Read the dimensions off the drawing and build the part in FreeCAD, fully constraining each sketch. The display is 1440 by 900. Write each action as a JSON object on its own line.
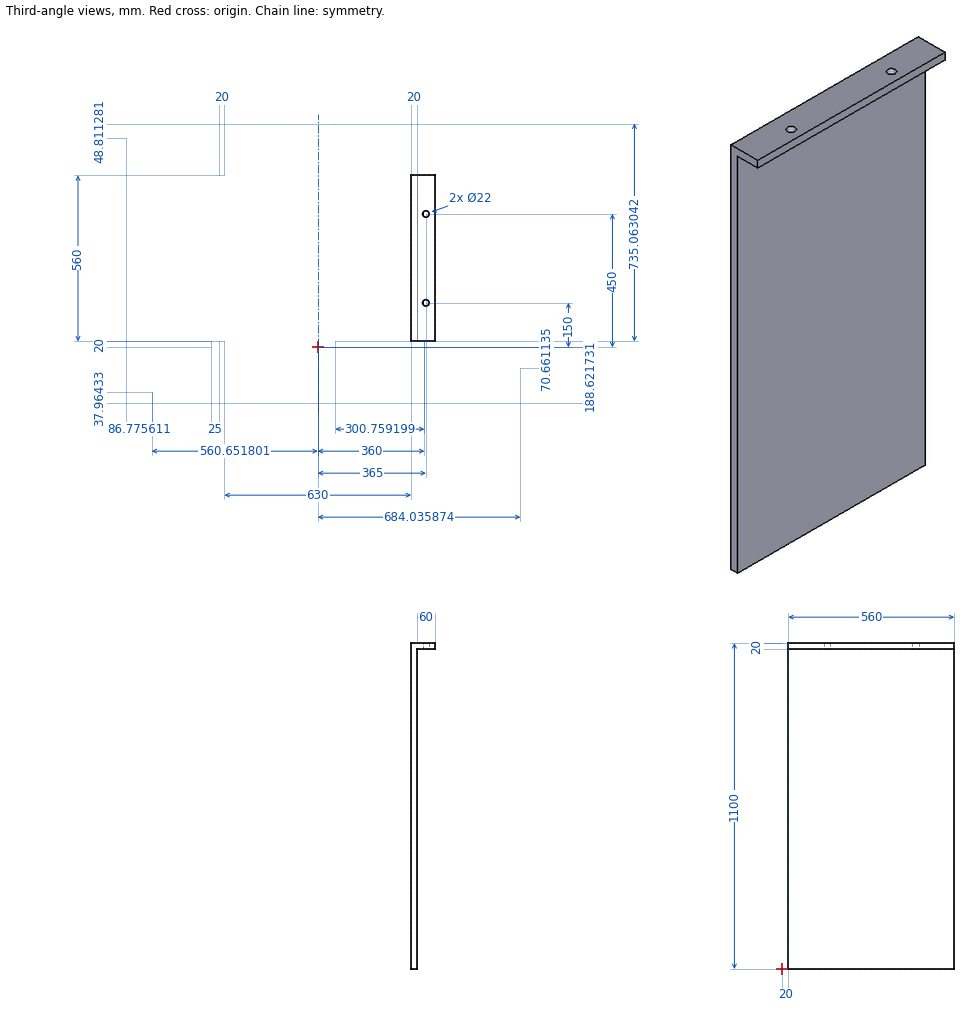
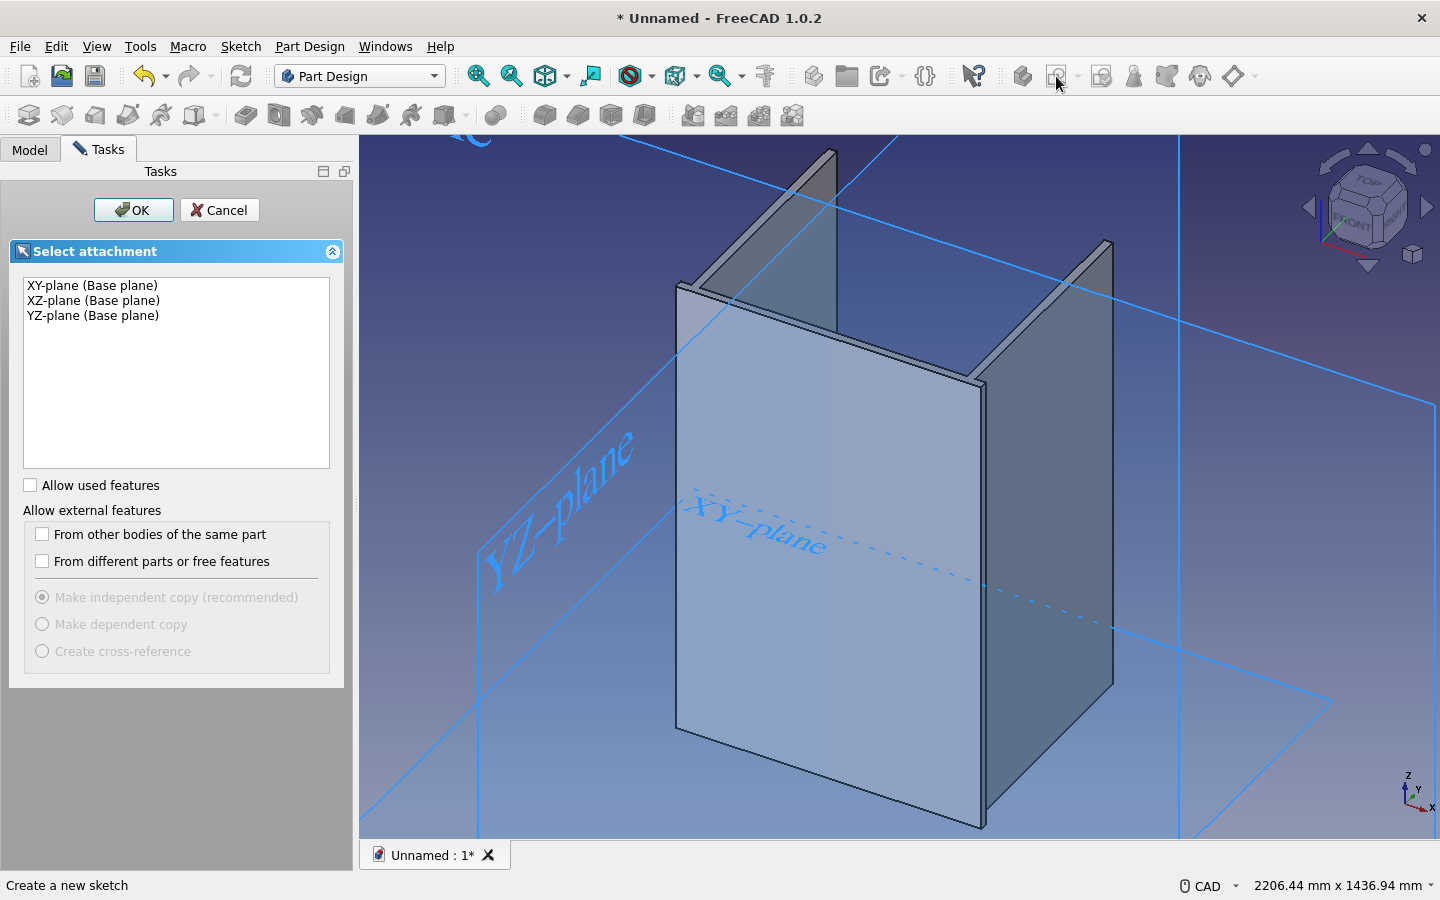
{"action": "left_click", "coordinate": [84, 286]}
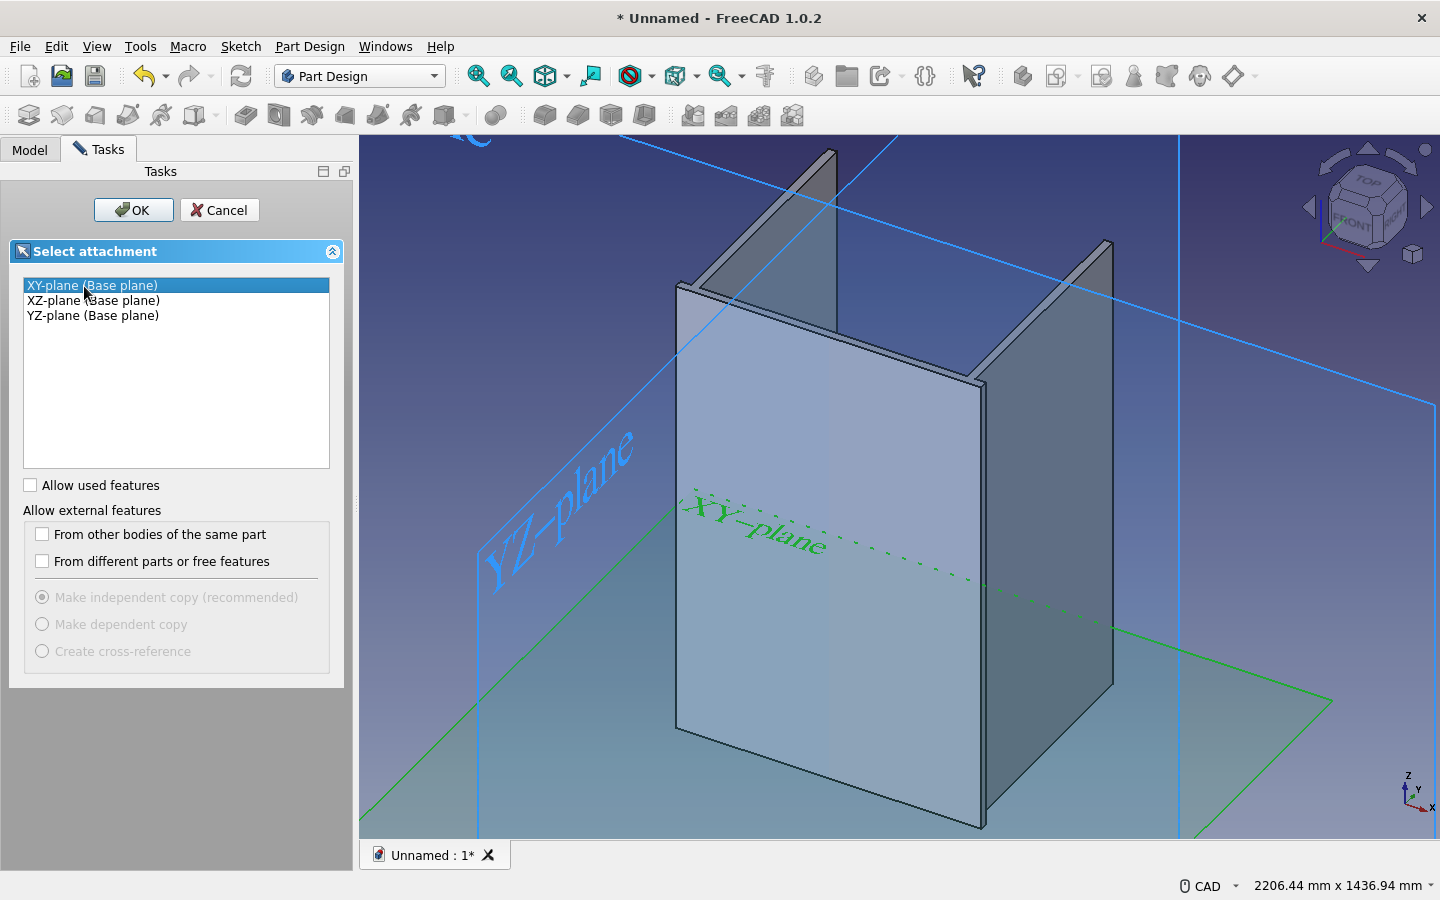
{"action": "left_click", "coordinate": [134, 210]}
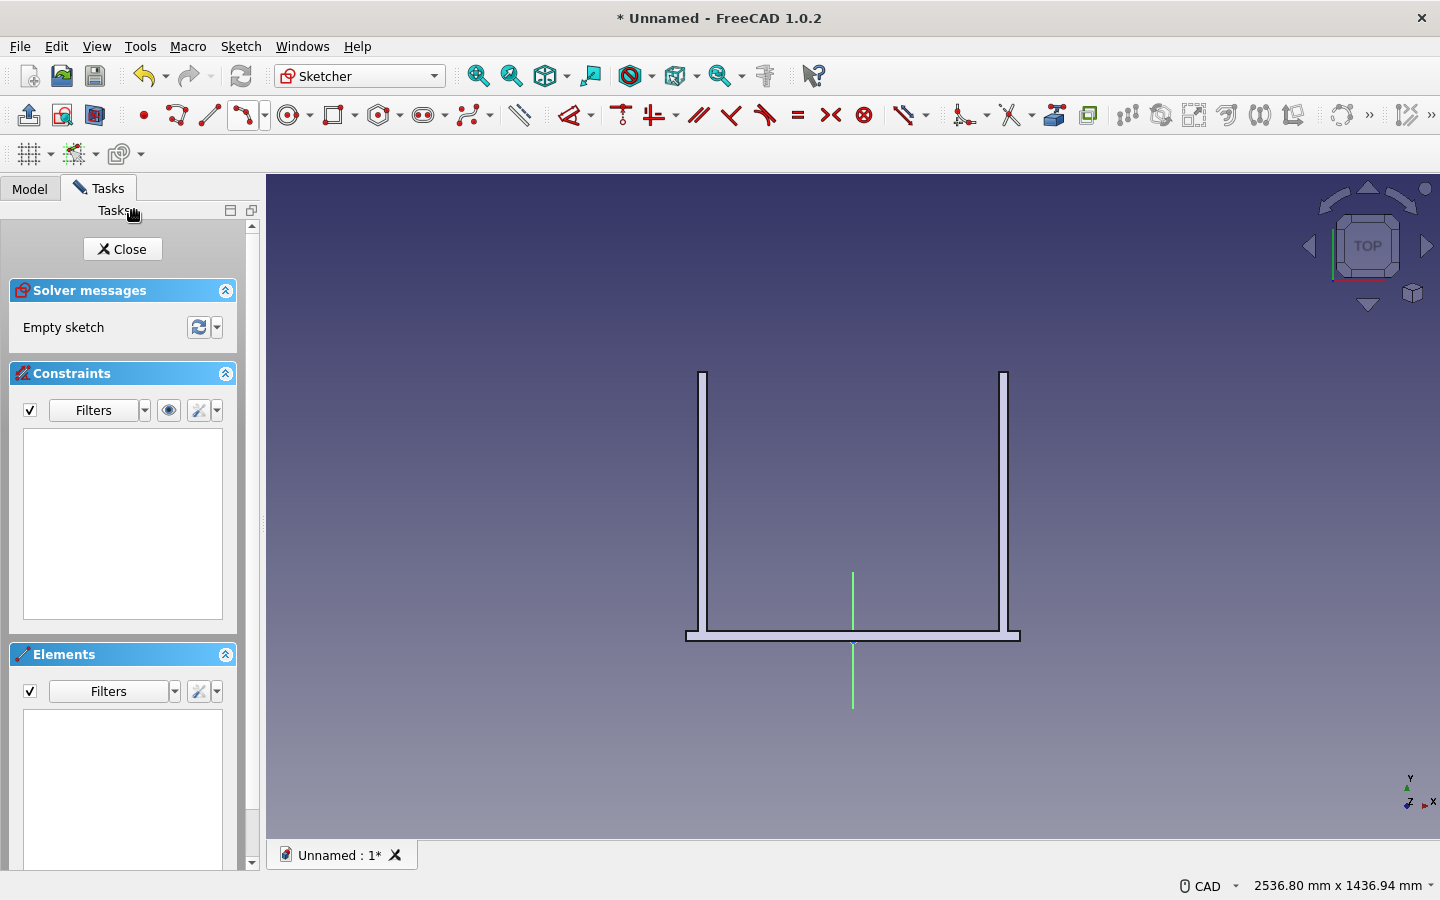
{"action": "left_click", "coordinate": [95, 116]}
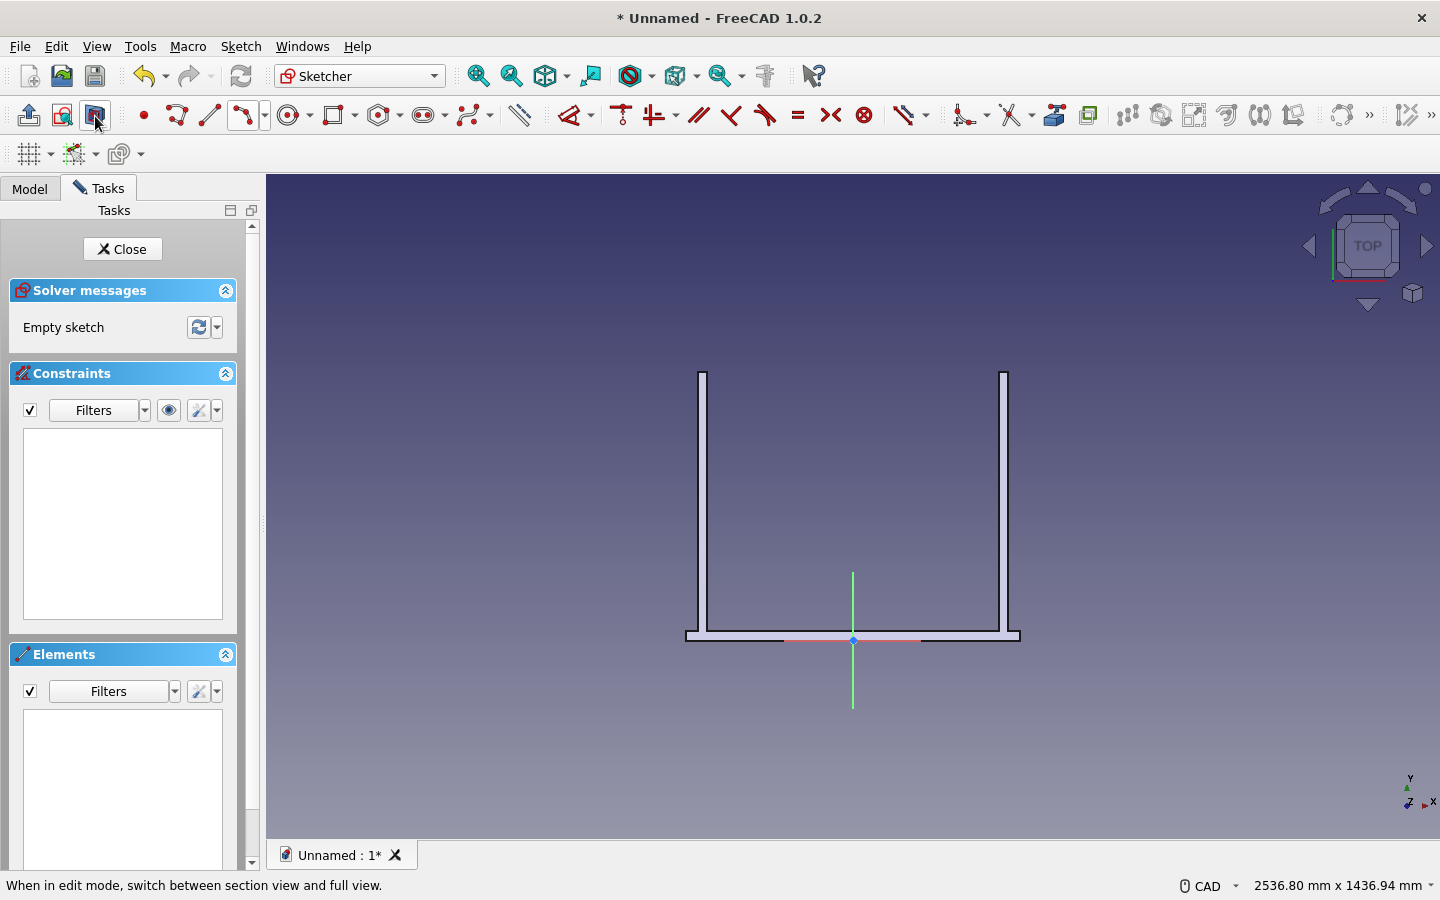
{"action": "left_click", "coordinate": [177, 116]}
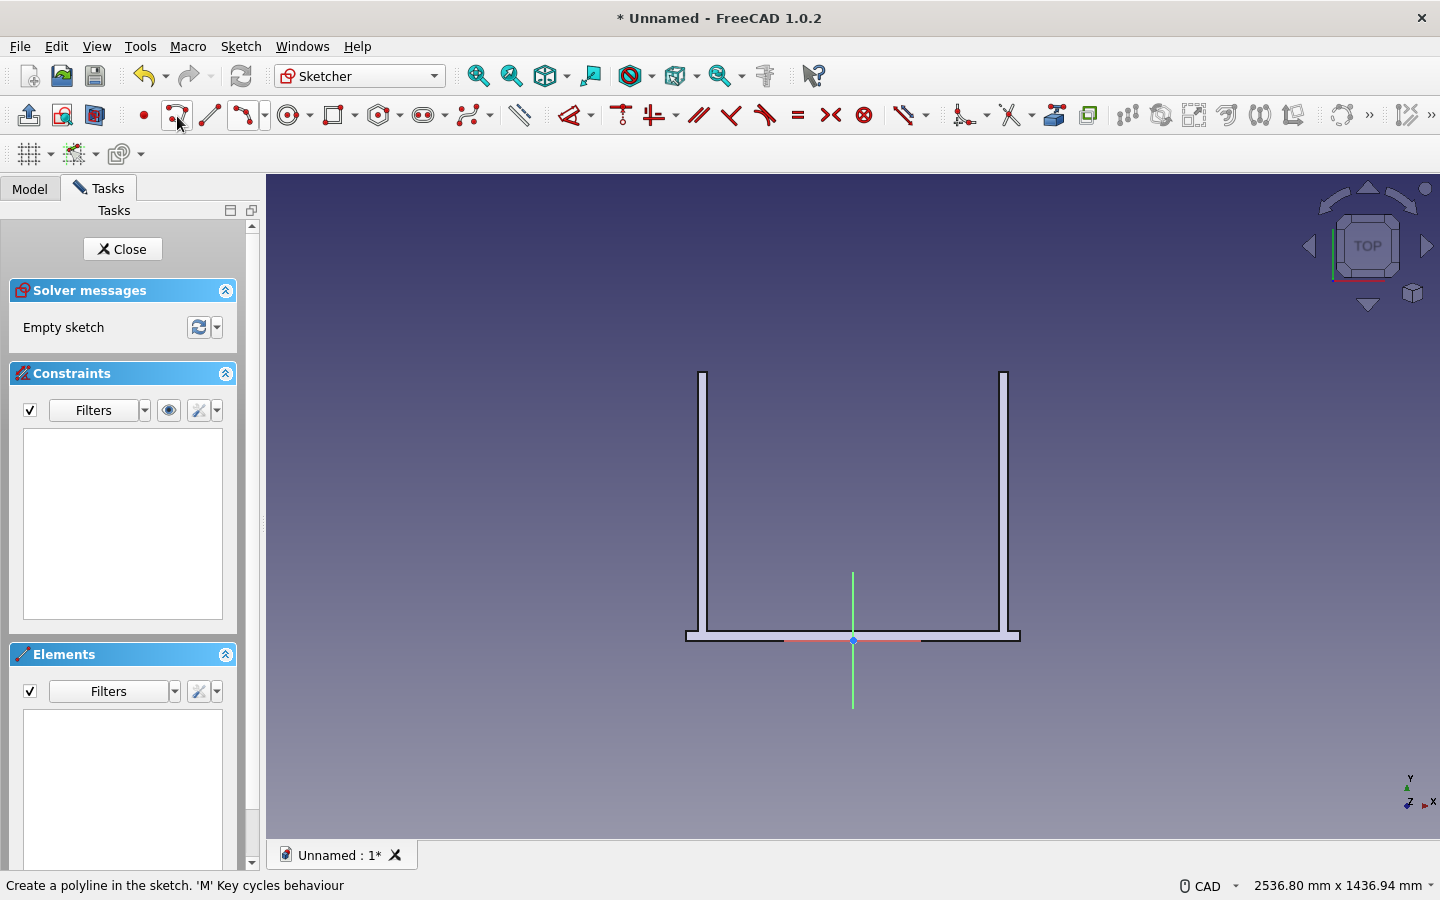
{"action": "scroll", "coordinate": [880, 631], "scroll_direction": "up", "scroll_amount": 3}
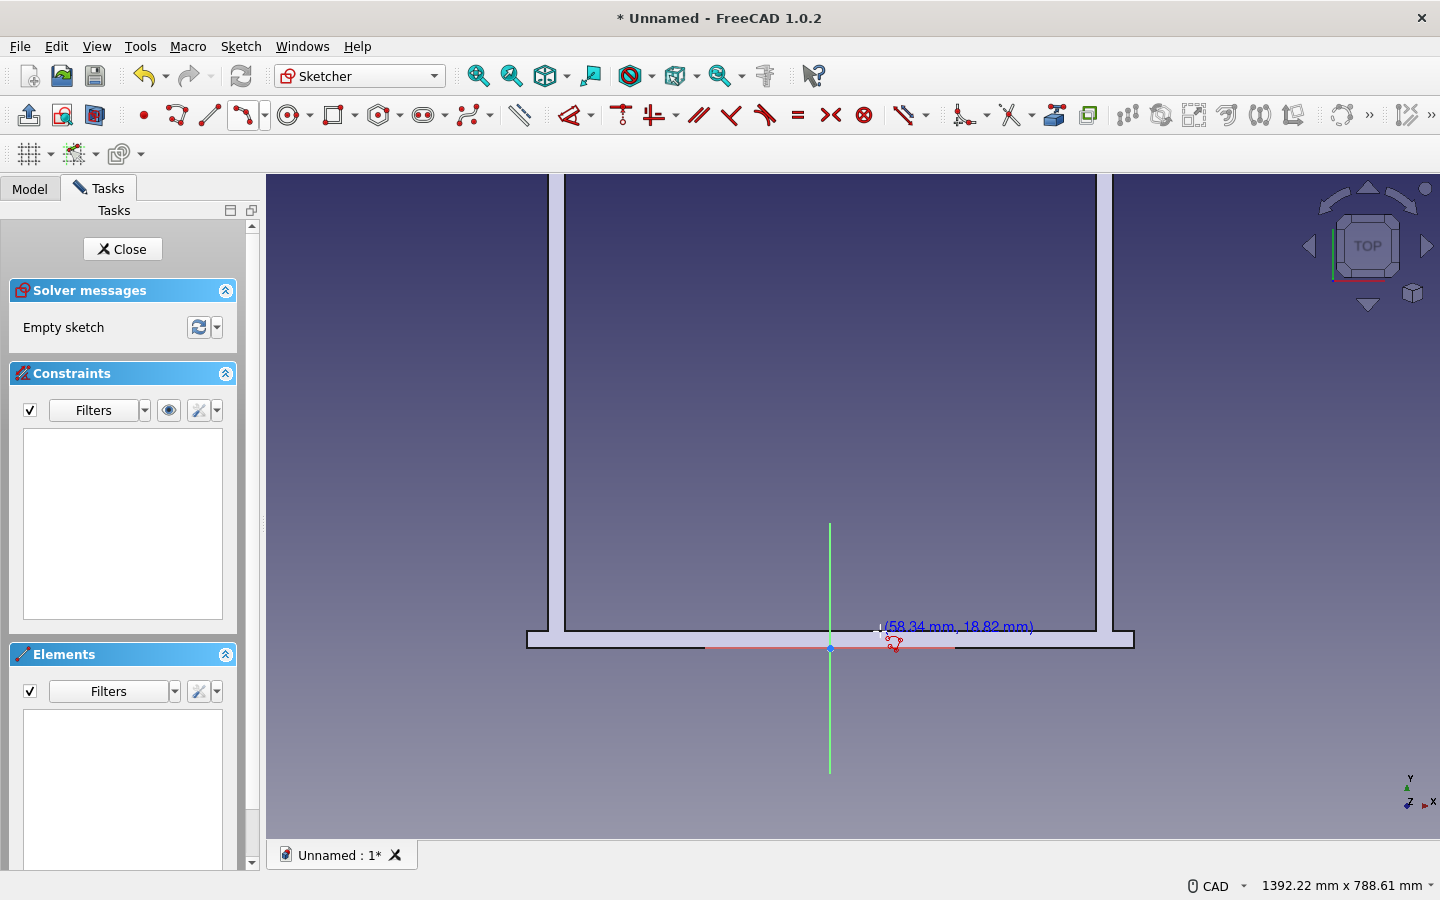
{"action": "left_click", "coordinate": [880, 631]}
{"action": "left_click", "coordinate": [1134, 631]}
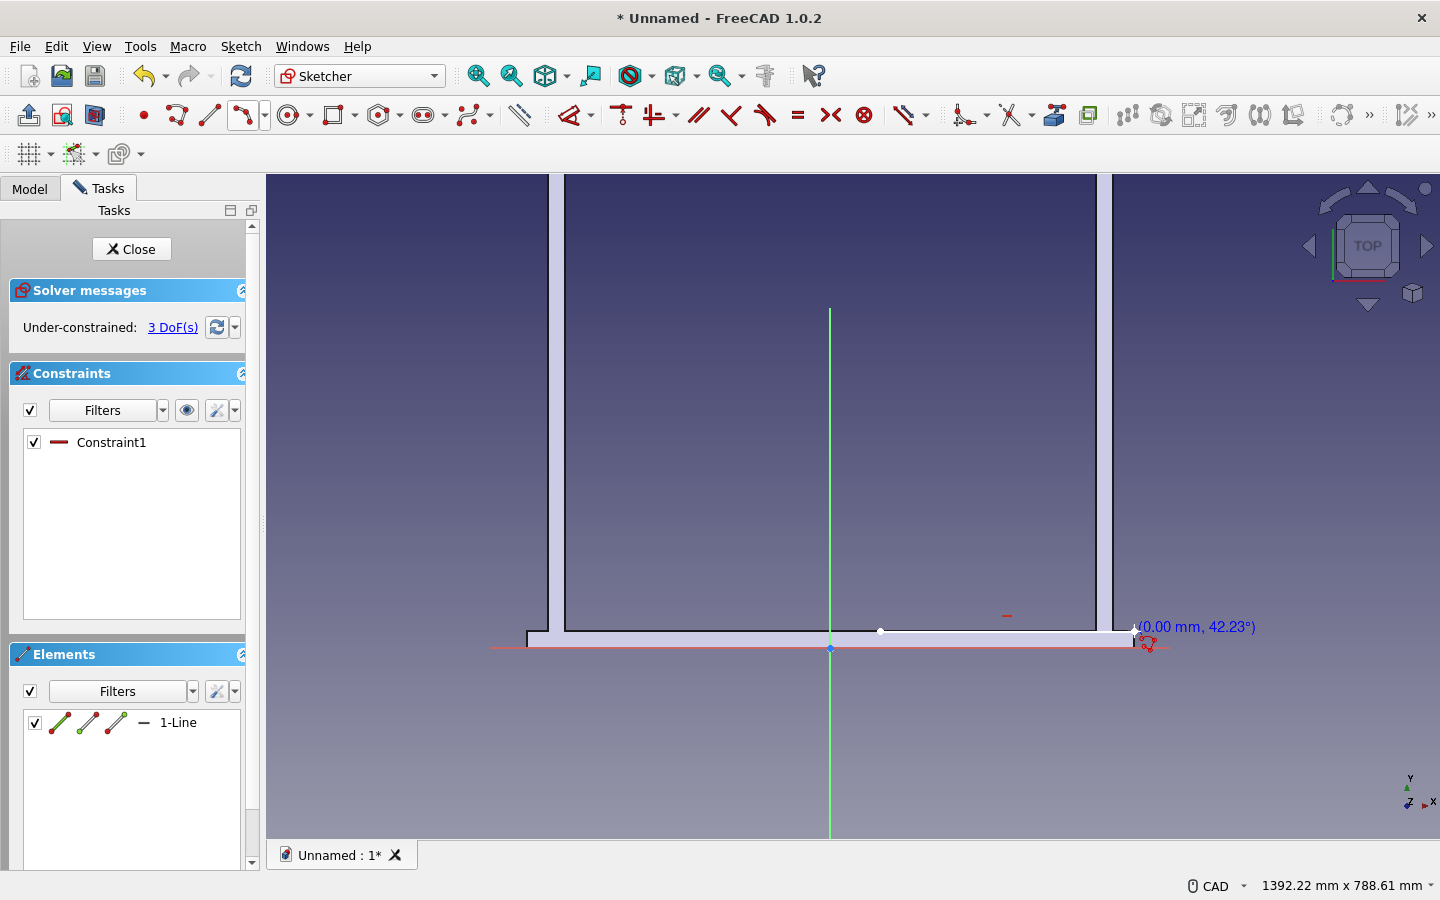
{"action": "scroll", "coordinate": [710, 625], "scroll_direction": "down", "scroll_amount": 3}